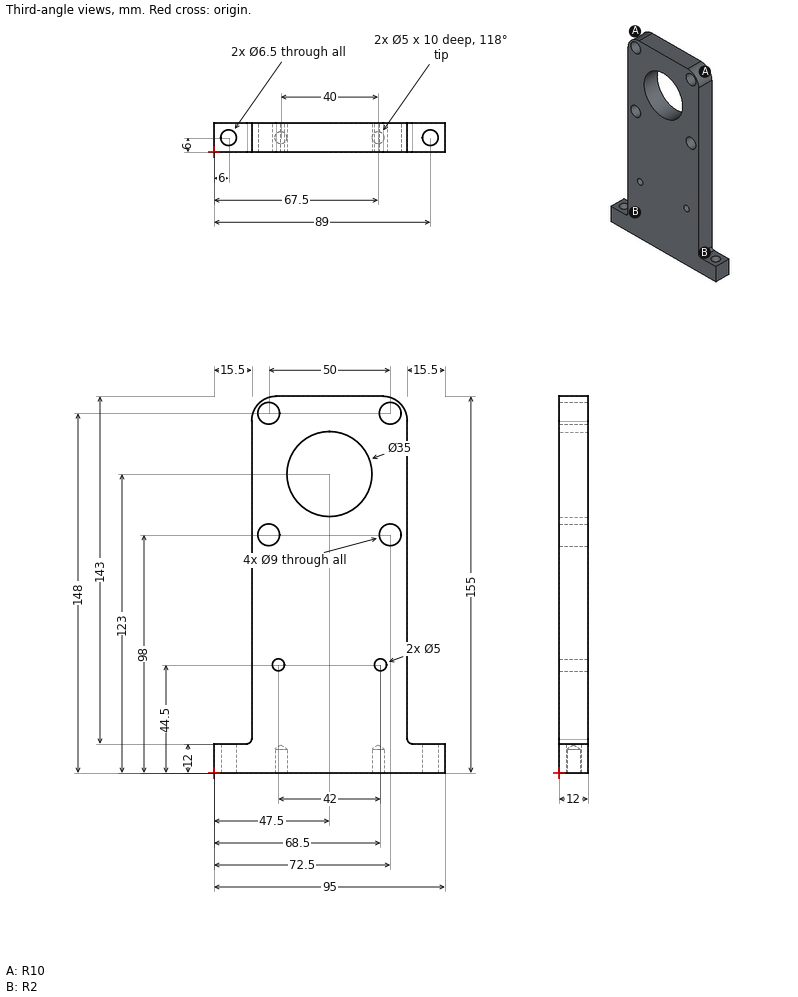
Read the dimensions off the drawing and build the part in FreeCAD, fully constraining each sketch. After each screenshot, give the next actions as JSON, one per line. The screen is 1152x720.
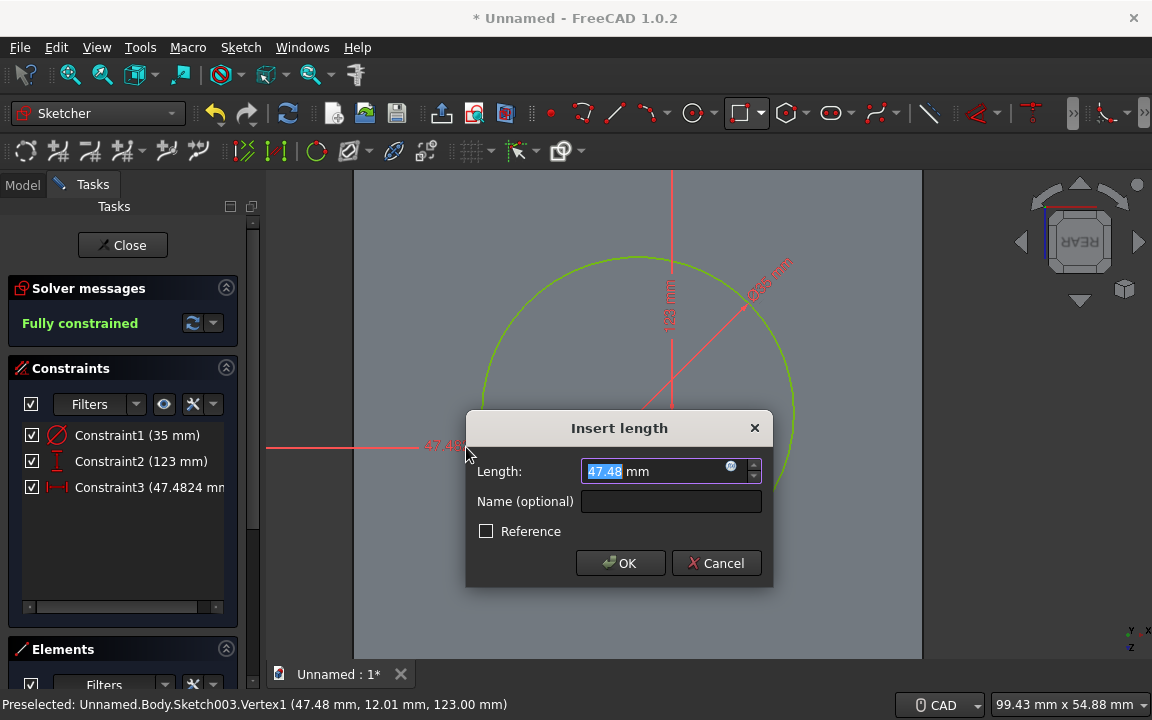
{"action": "type", "text": "47.5"}
{"action": "key", "text": "Return"}
{"action": "key", "text": "Escape"}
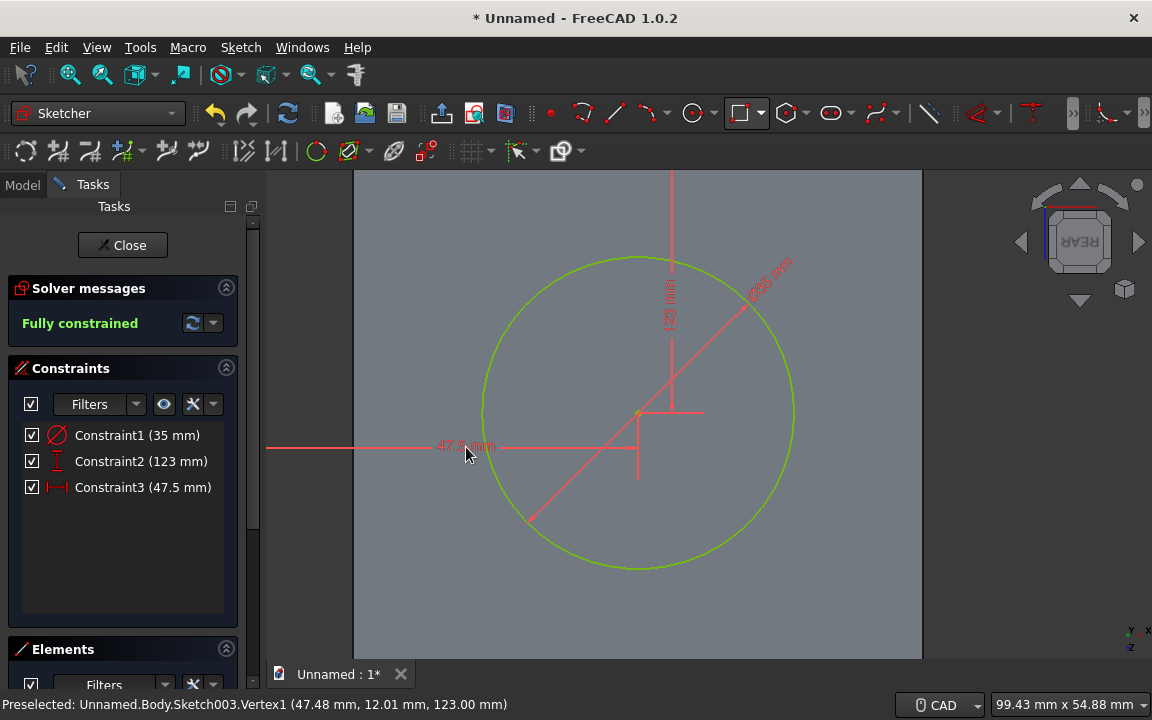
{"action": "left_click", "coordinate": [123, 245]}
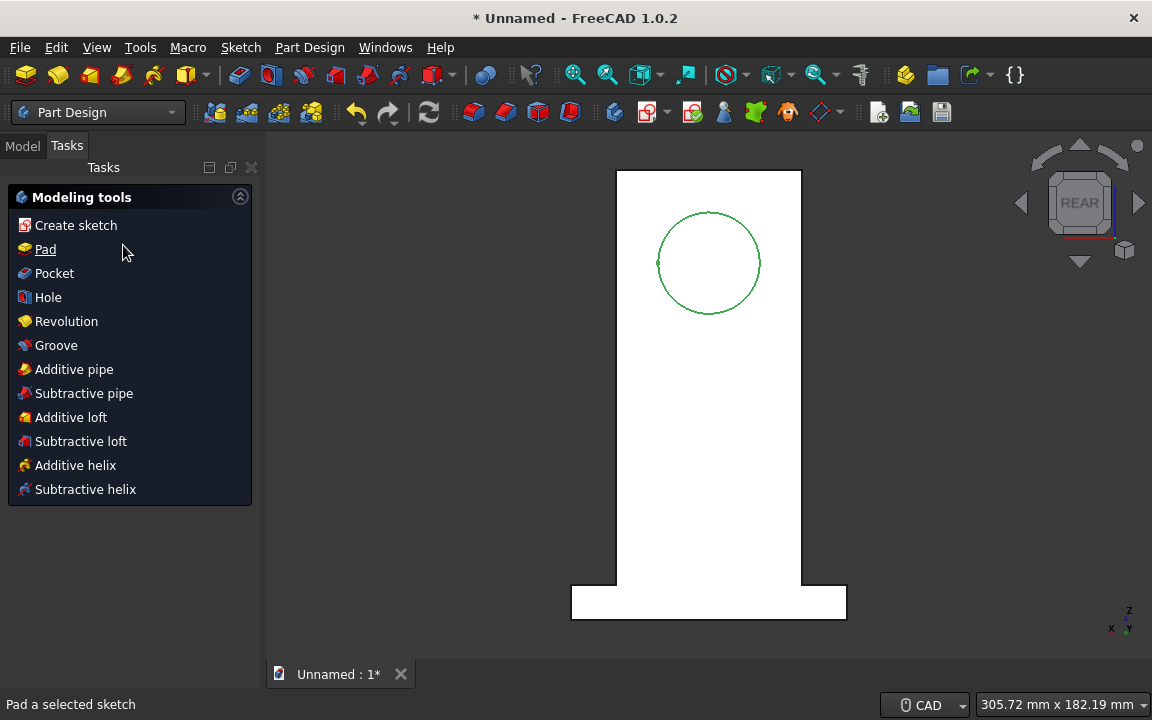
{"action": "left_click", "coordinate": [240, 76]}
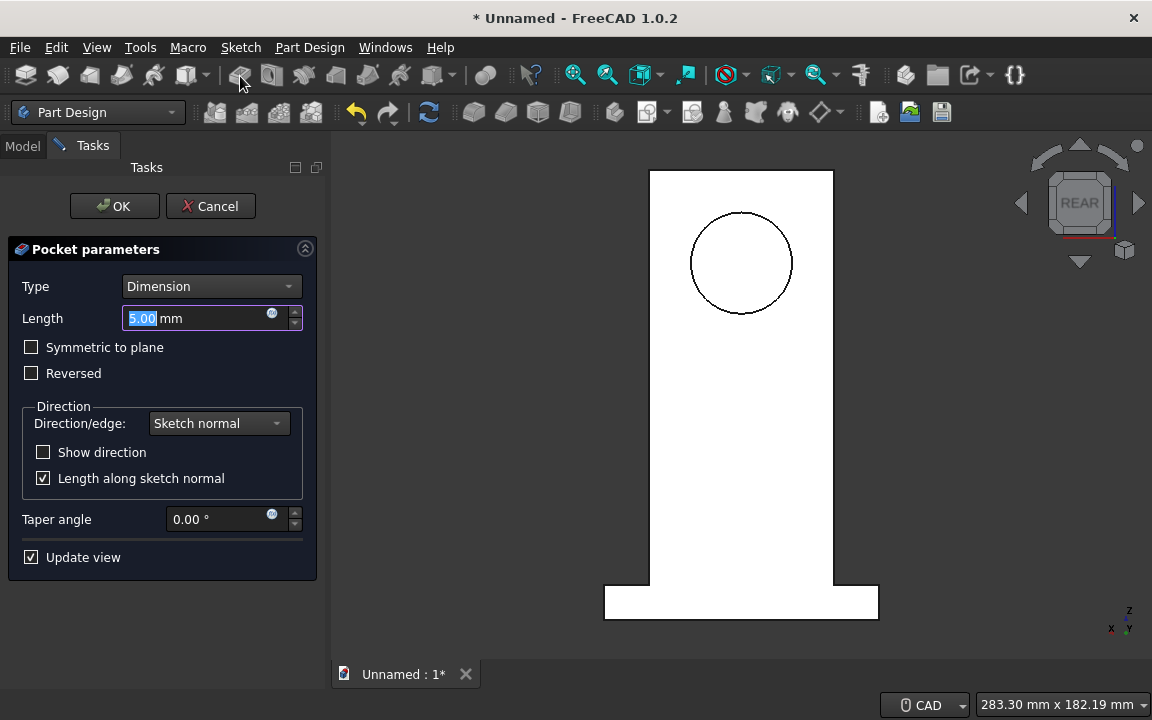
{"action": "left_click", "coordinate": [212, 286]}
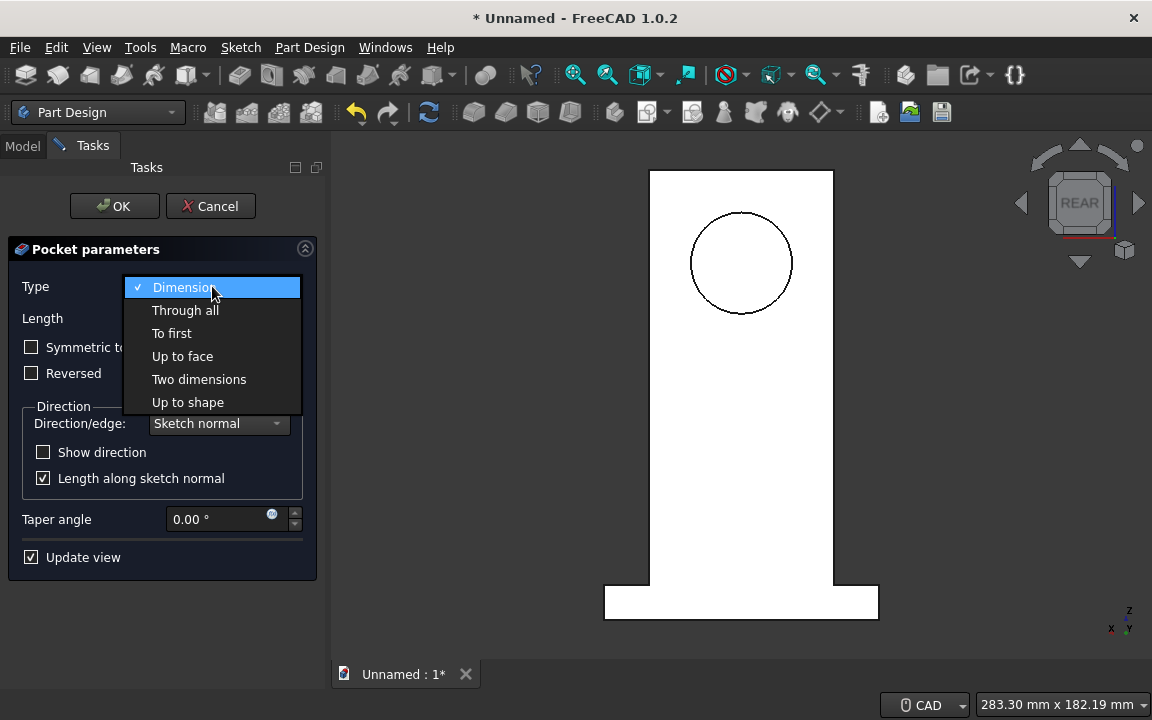
{"action": "left_click", "coordinate": [212, 310]}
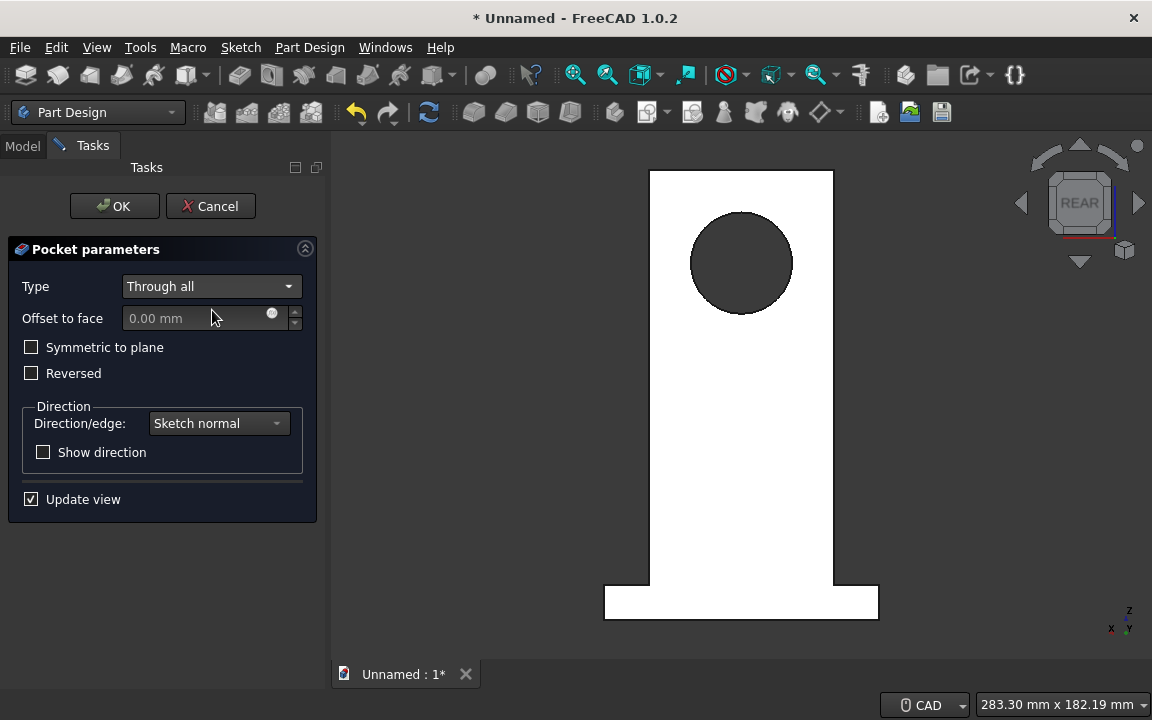
{"action": "left_click", "coordinate": [115, 206]}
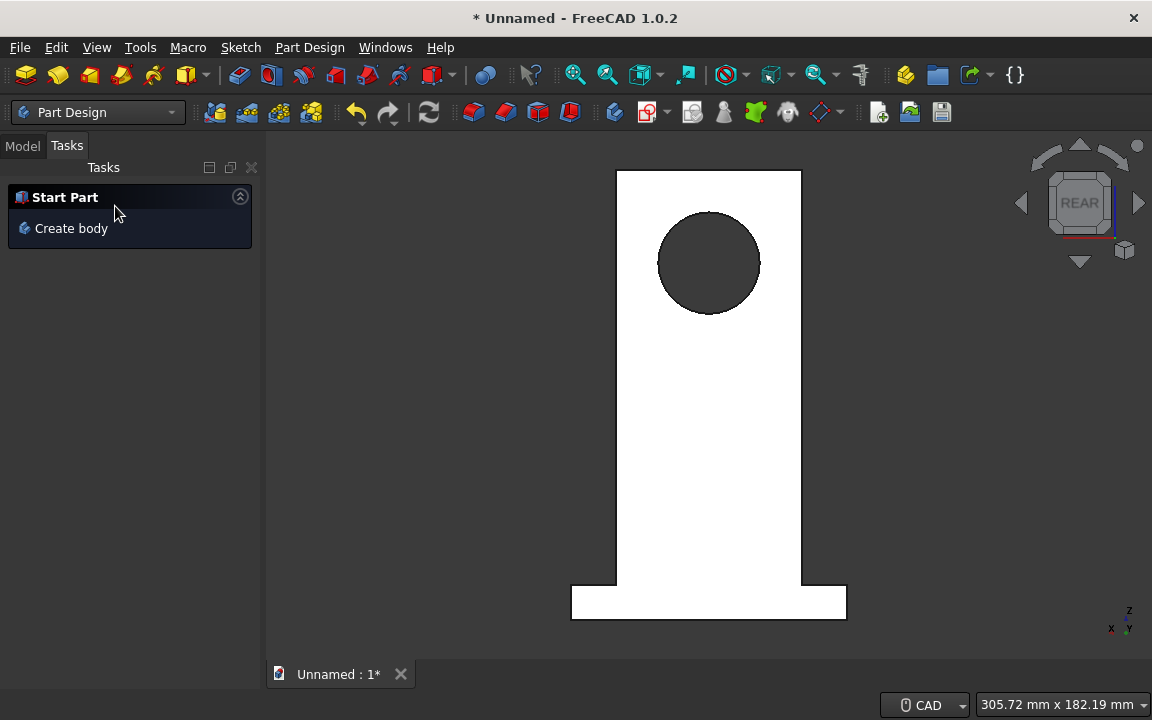
{"action": "key", "text": "0"}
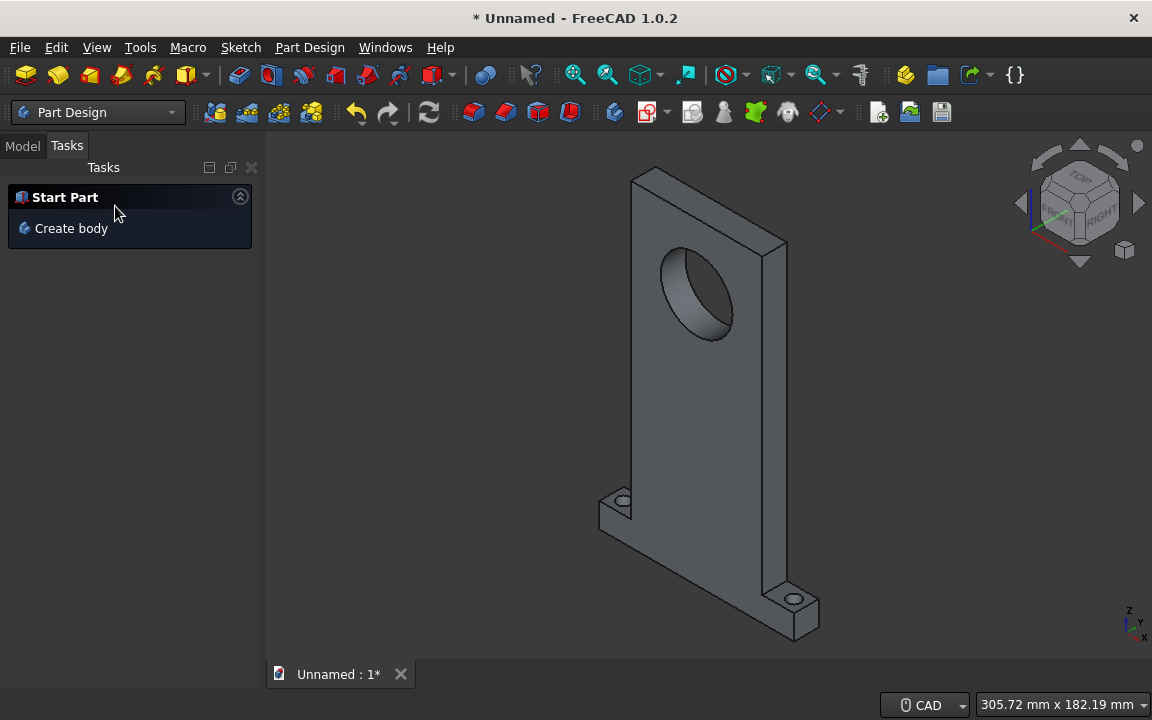
{"action": "left_click", "coordinate": [775, 248]}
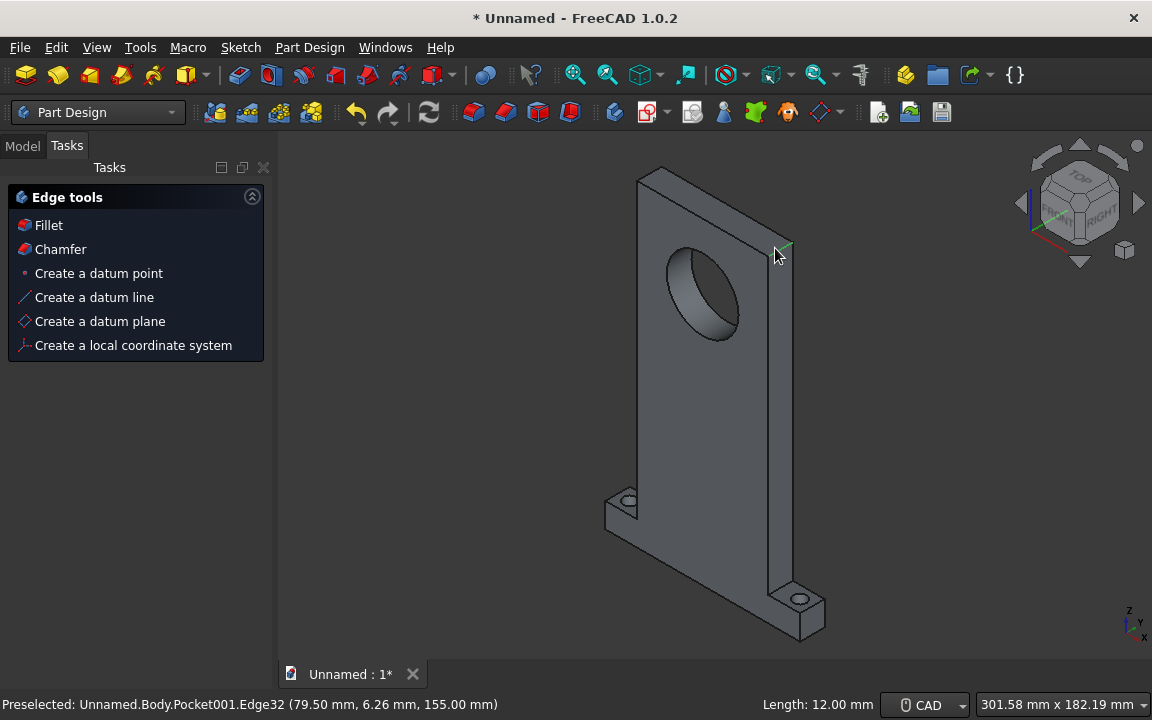
{"action": "key", "text": "2"}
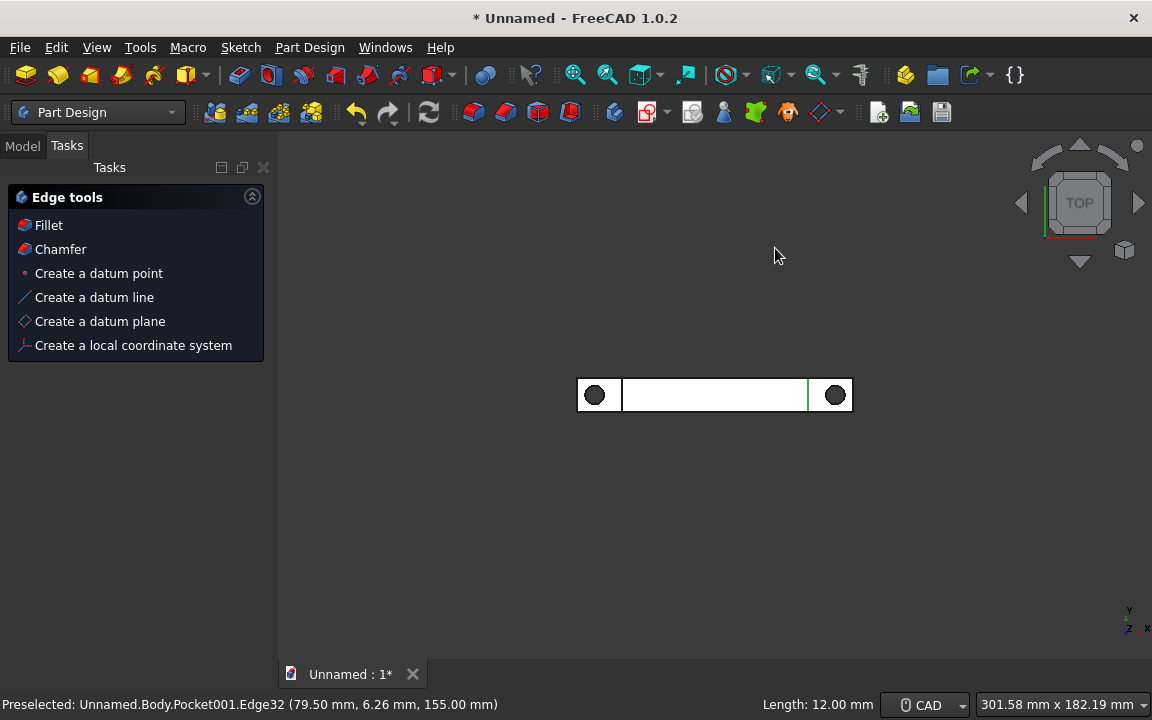
{"action": "left_click", "coordinate": [576, 76]}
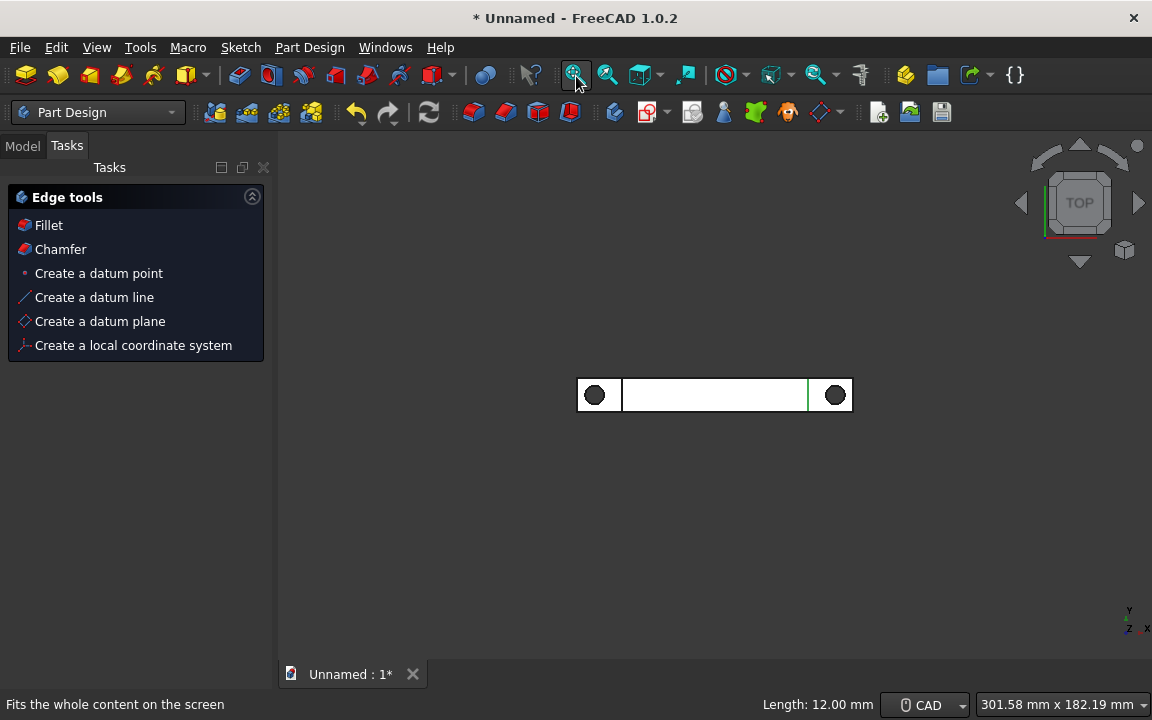
{"action": "left_click", "coordinate": [622, 394], "text": "ctrl"}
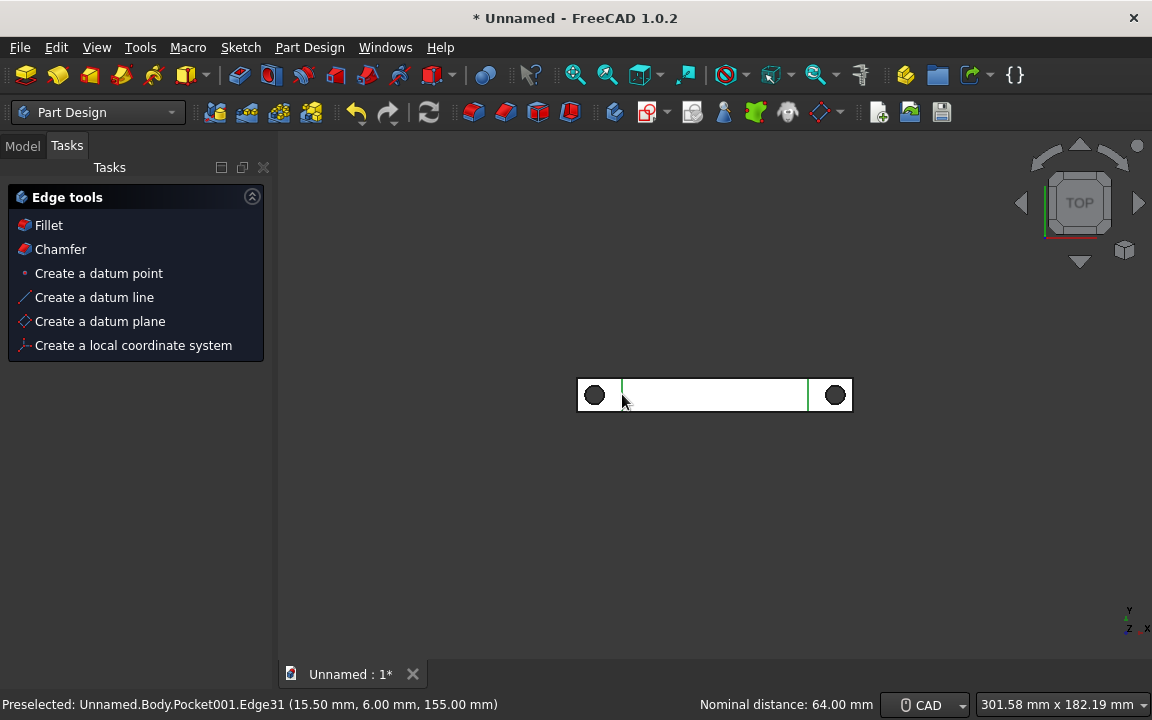
{"action": "left_click", "coordinate": [474, 112]}